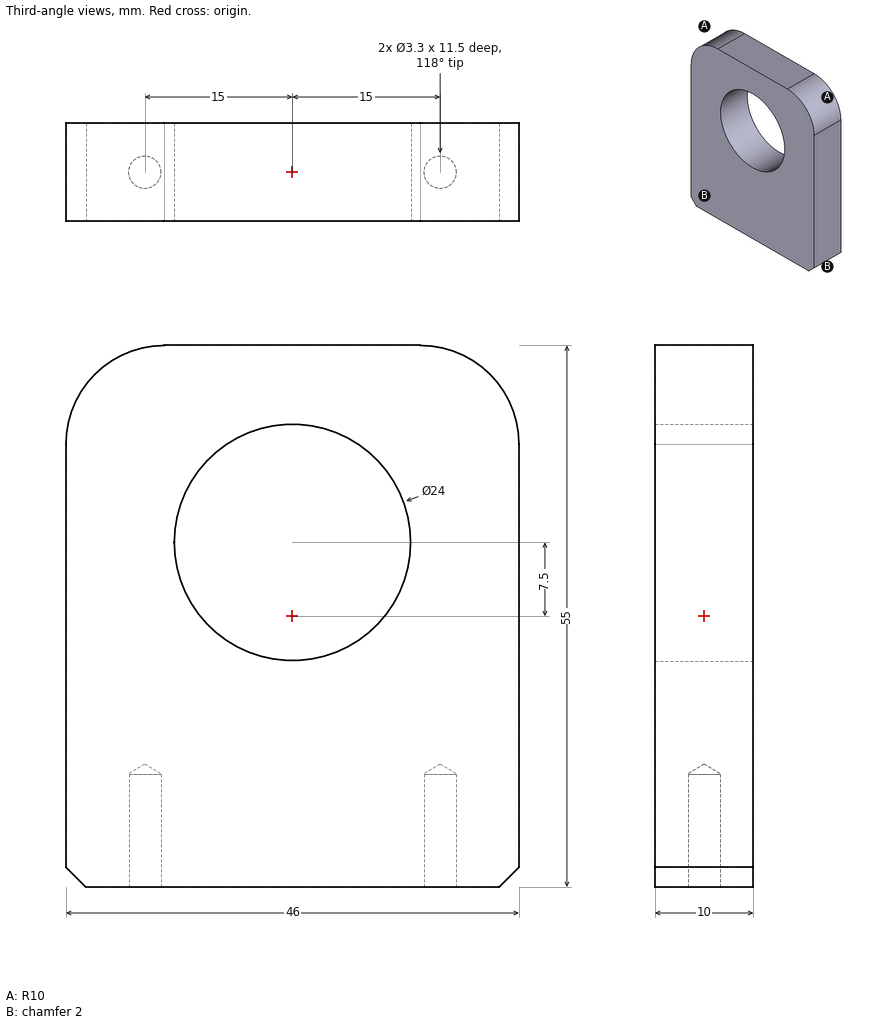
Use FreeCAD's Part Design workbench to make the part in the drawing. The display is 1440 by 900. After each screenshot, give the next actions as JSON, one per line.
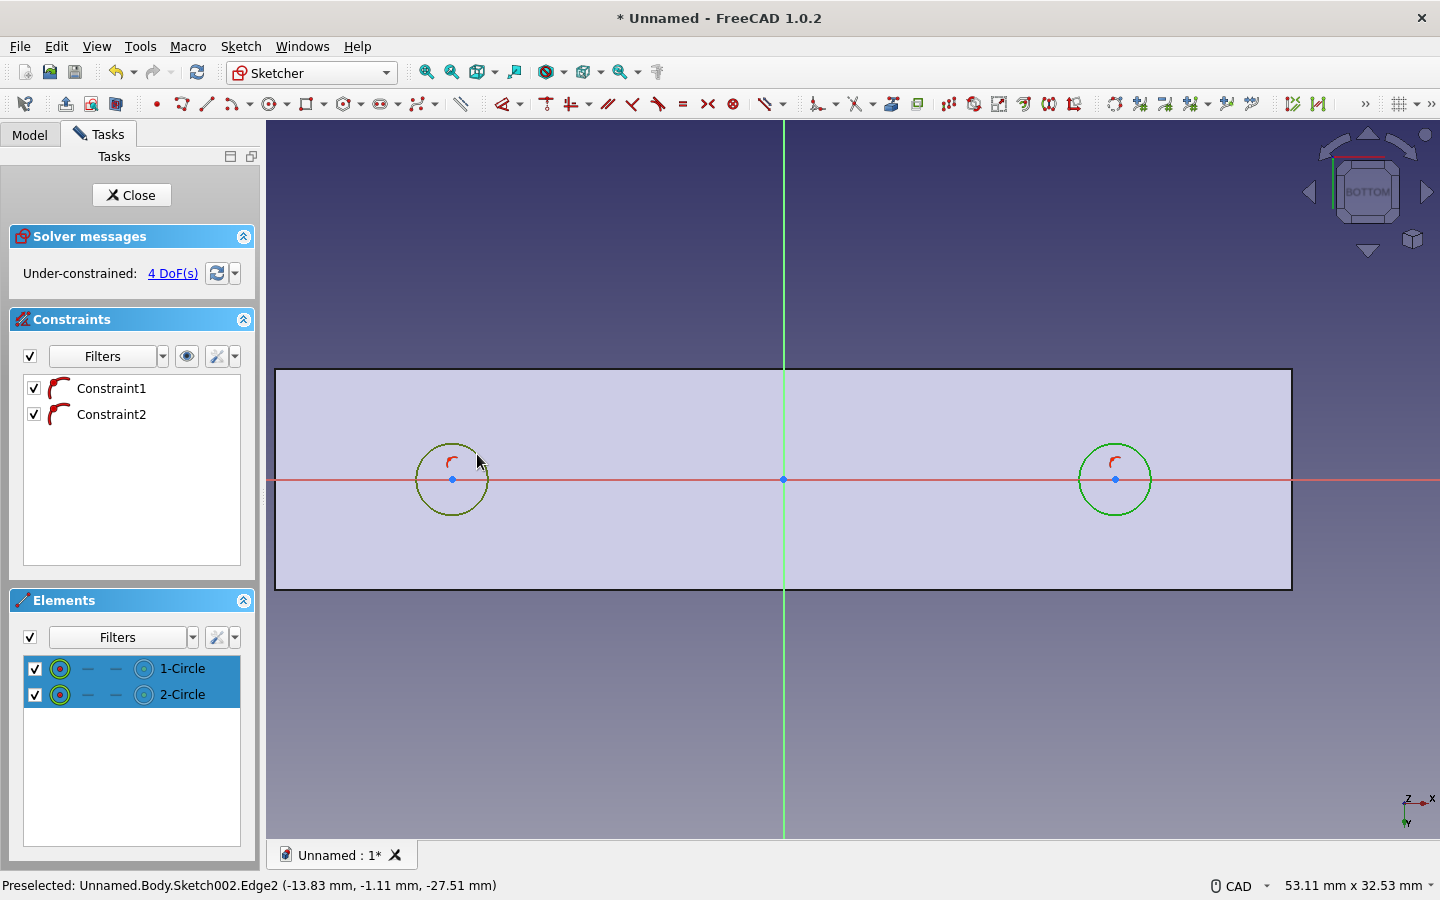
{"action": "left_click", "coordinate": [683, 104]}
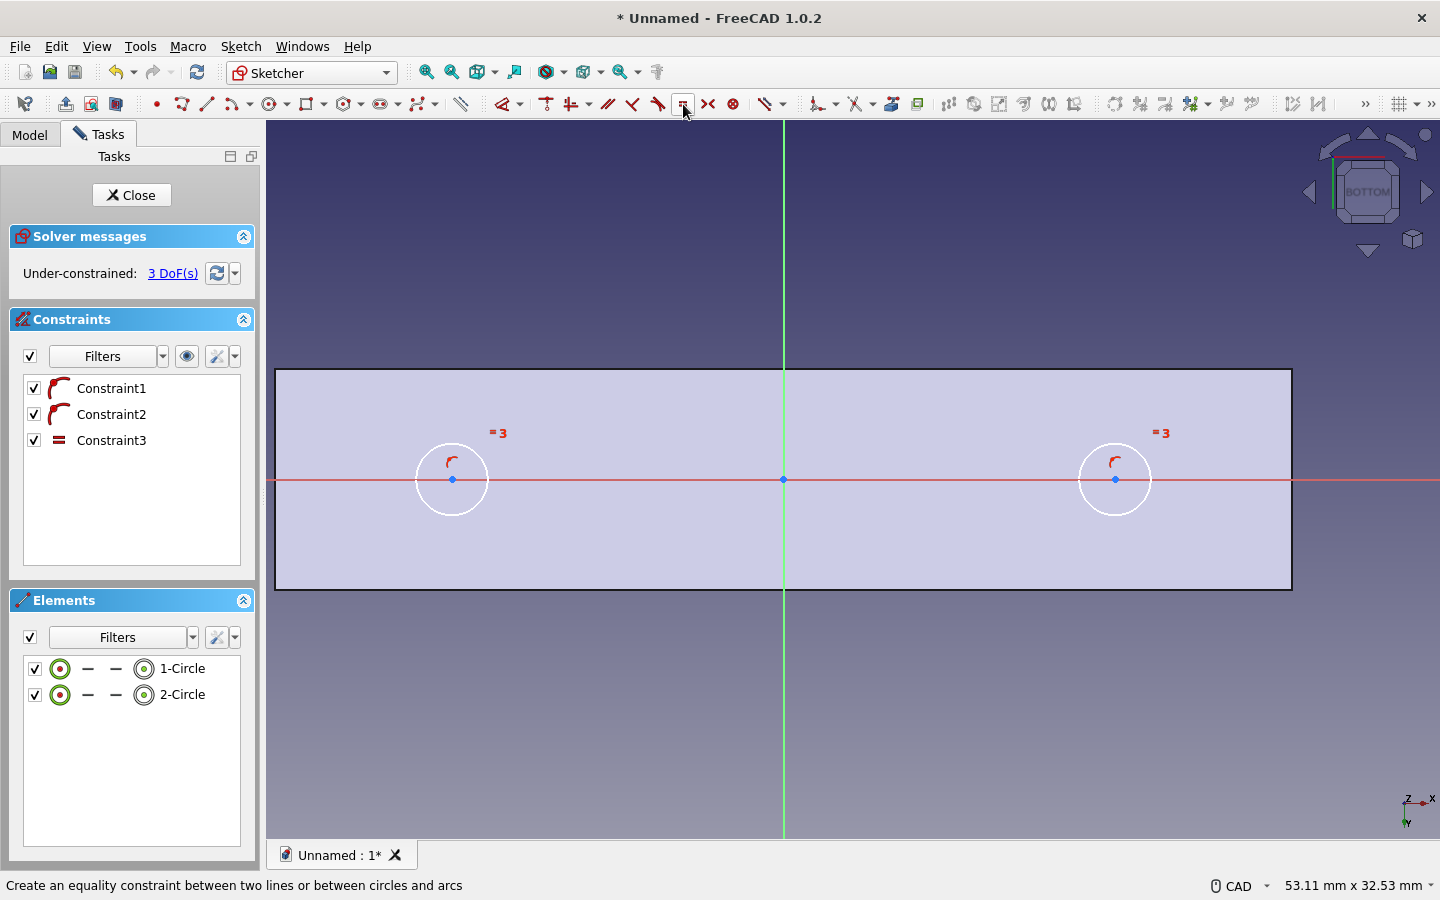
{"action": "left_click", "coordinate": [502, 104]}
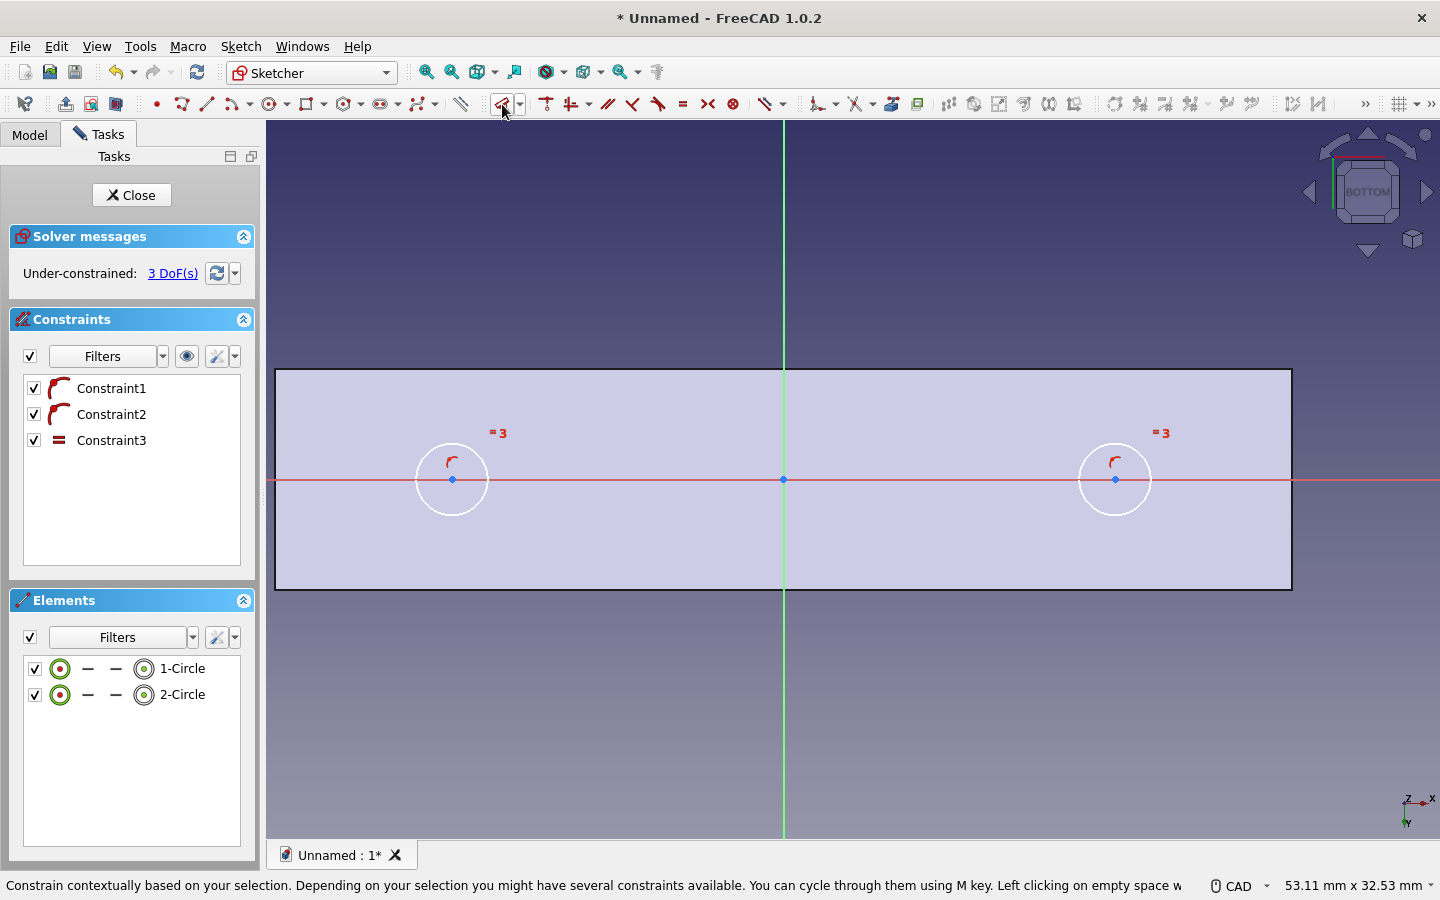
{"action": "left_click", "coordinate": [1140, 454]}
{"action": "left_click", "coordinate": [1162, 431]}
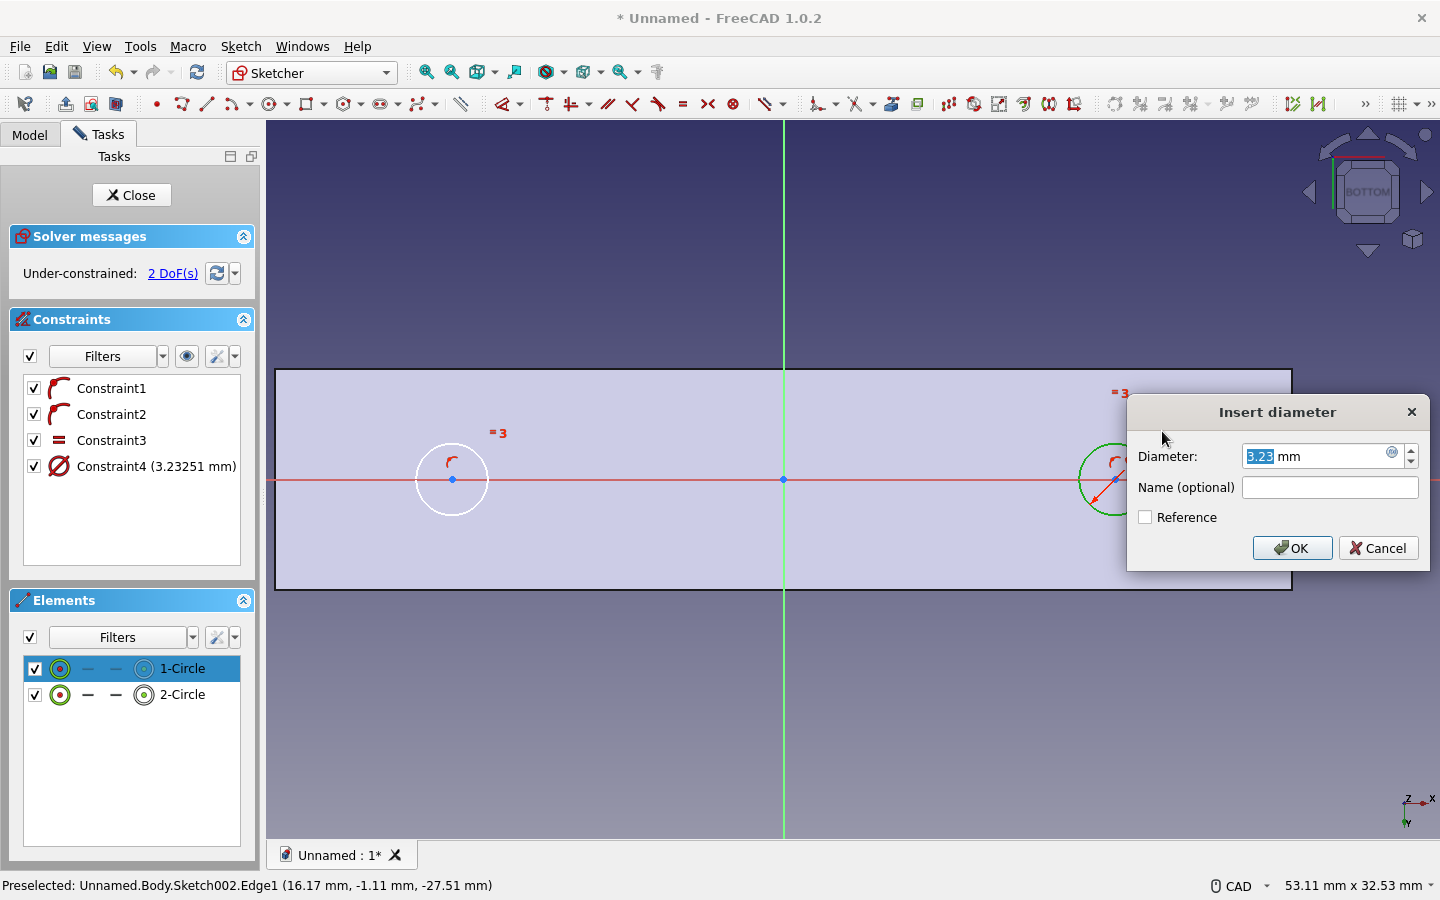
{"action": "type", "text": "3.3"}
{"action": "key", "text": "Return"}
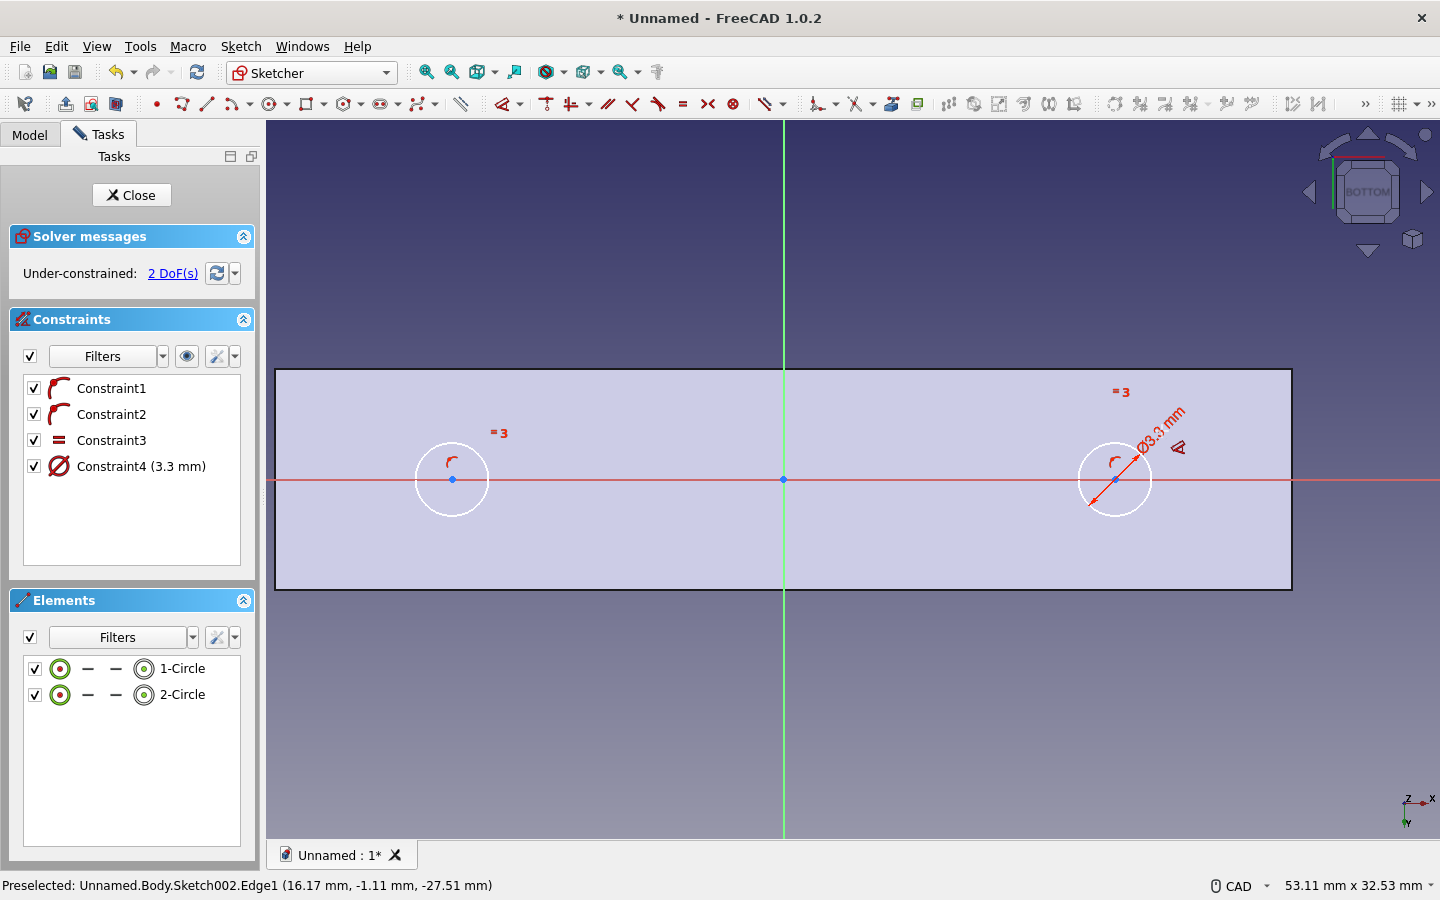
{"action": "left_click", "coordinate": [1115, 479]}
{"action": "left_click", "coordinate": [949, 513]}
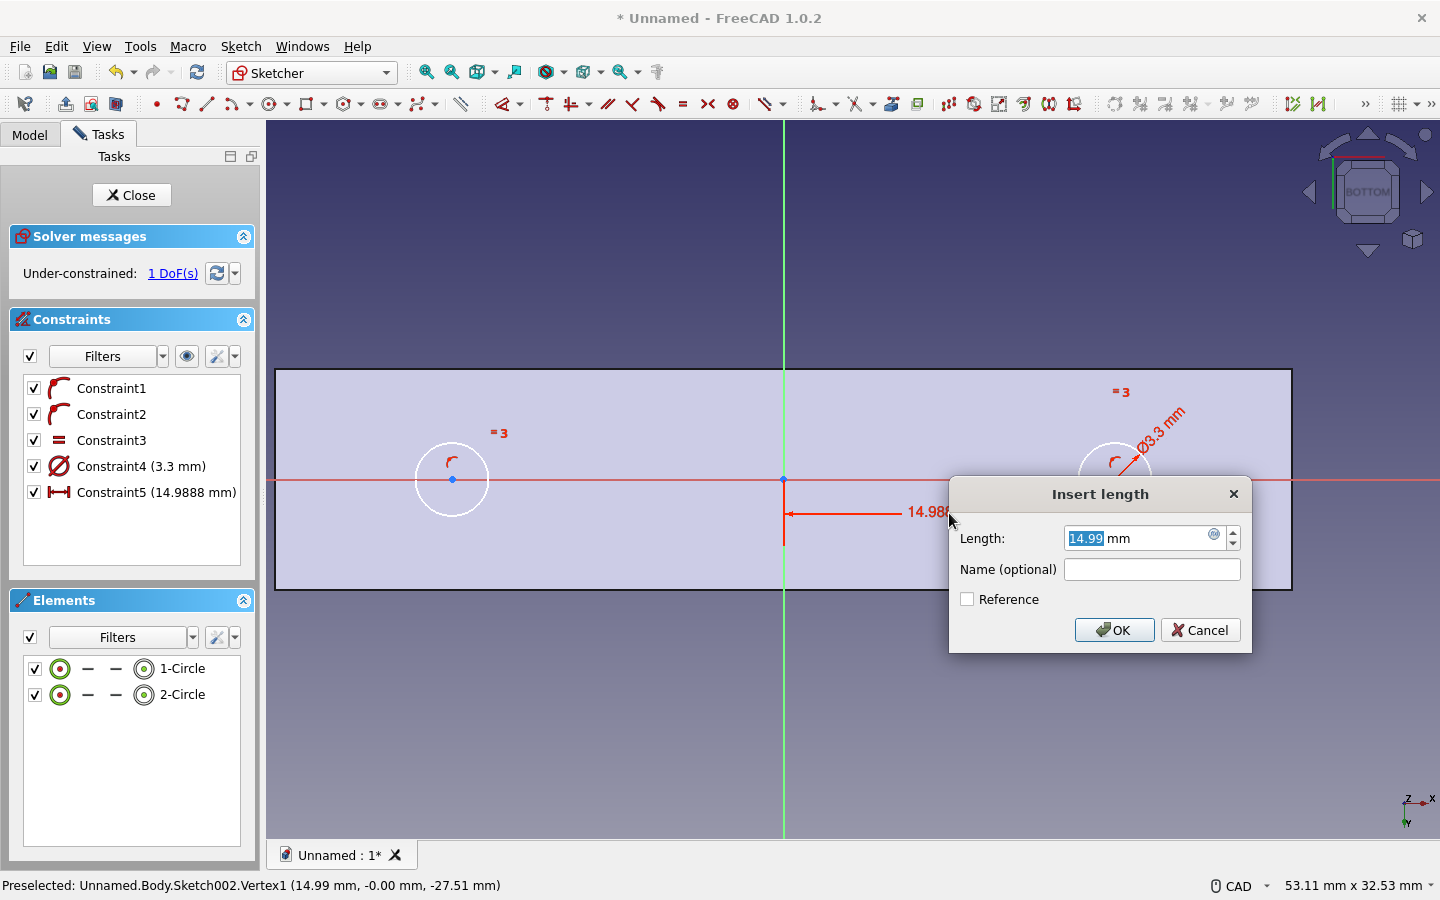
{"action": "type", "text": "15"}
{"action": "key", "text": "Return"}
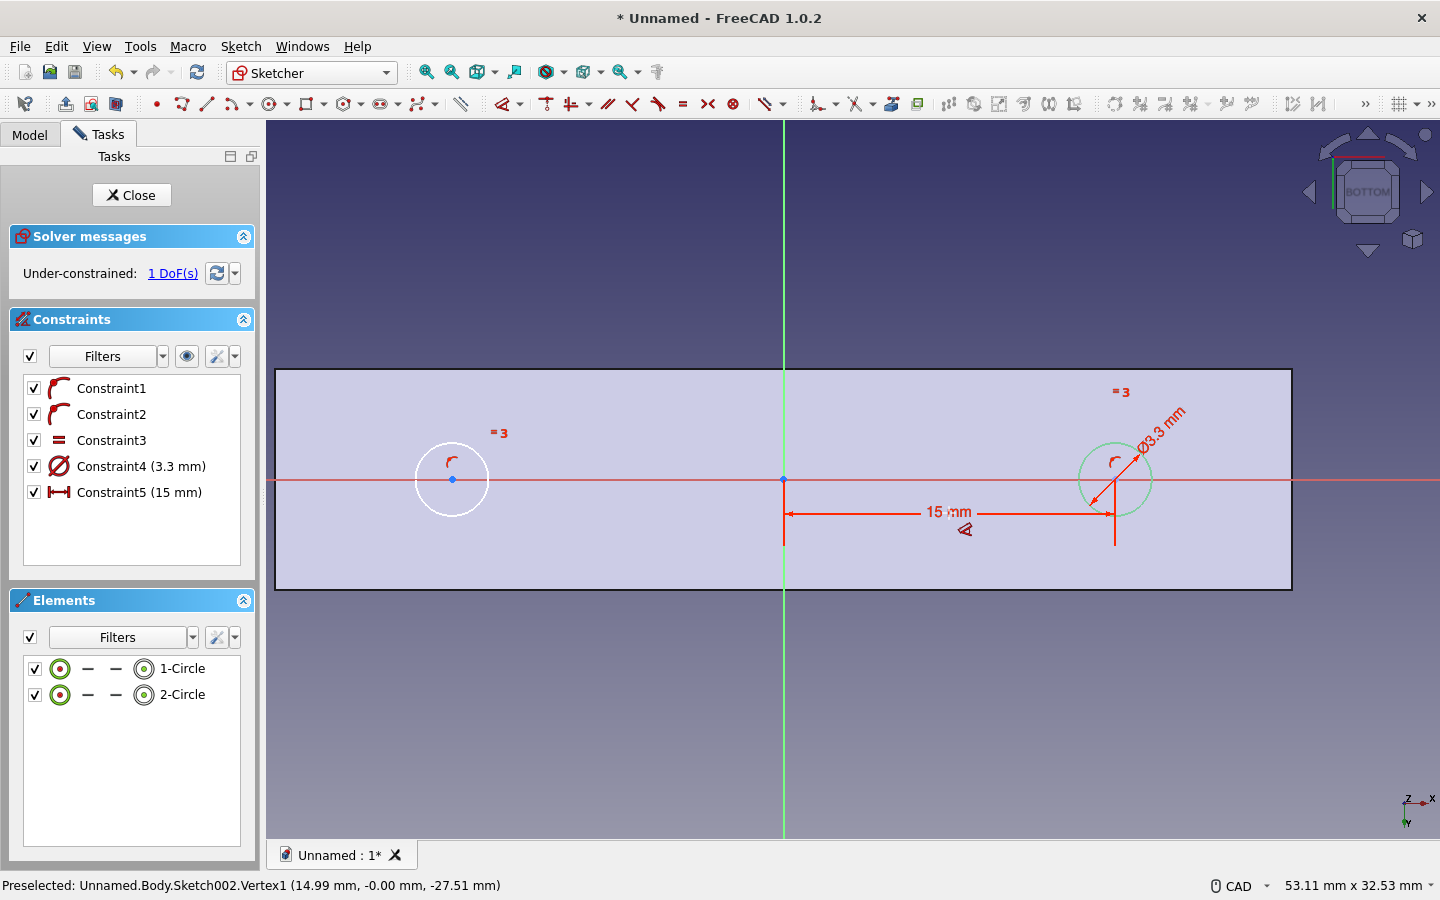
{"action": "left_click", "coordinate": [452, 479]}
{"action": "left_click", "coordinate": [618, 513]}